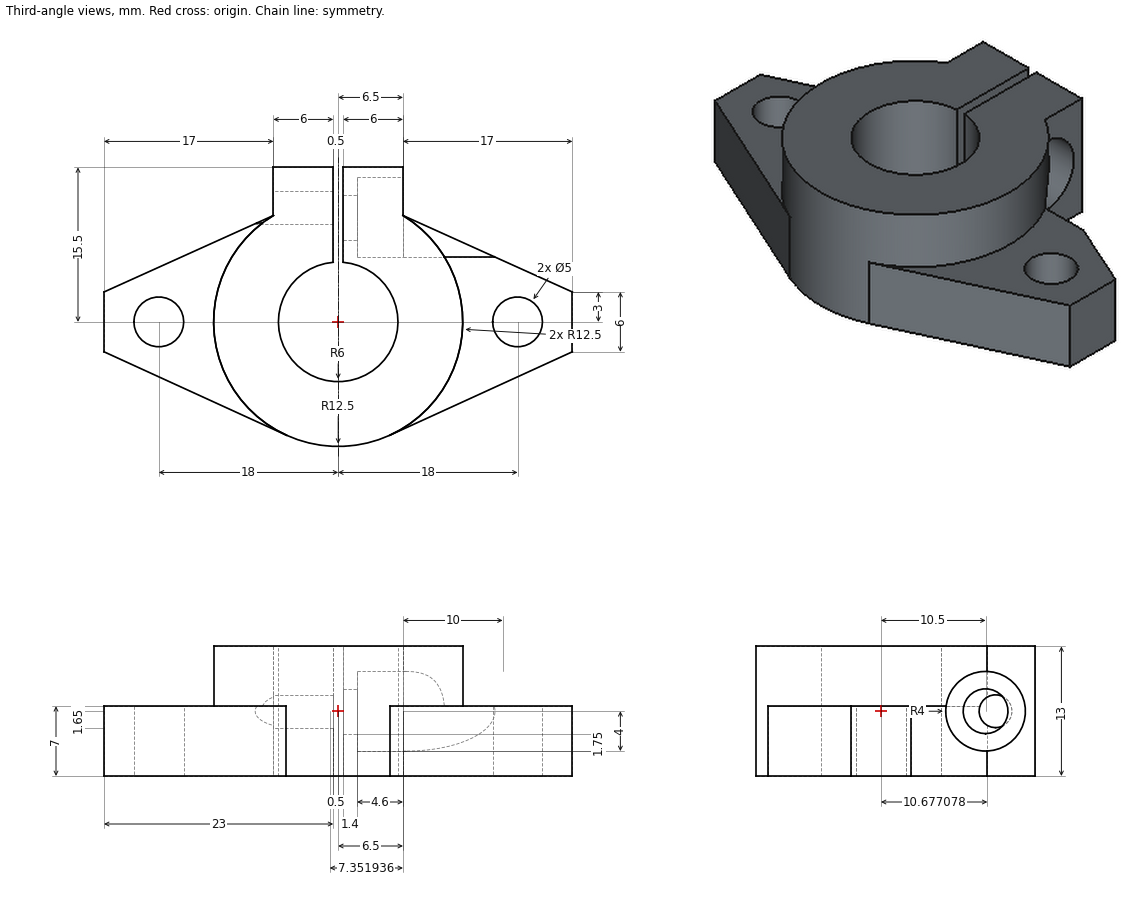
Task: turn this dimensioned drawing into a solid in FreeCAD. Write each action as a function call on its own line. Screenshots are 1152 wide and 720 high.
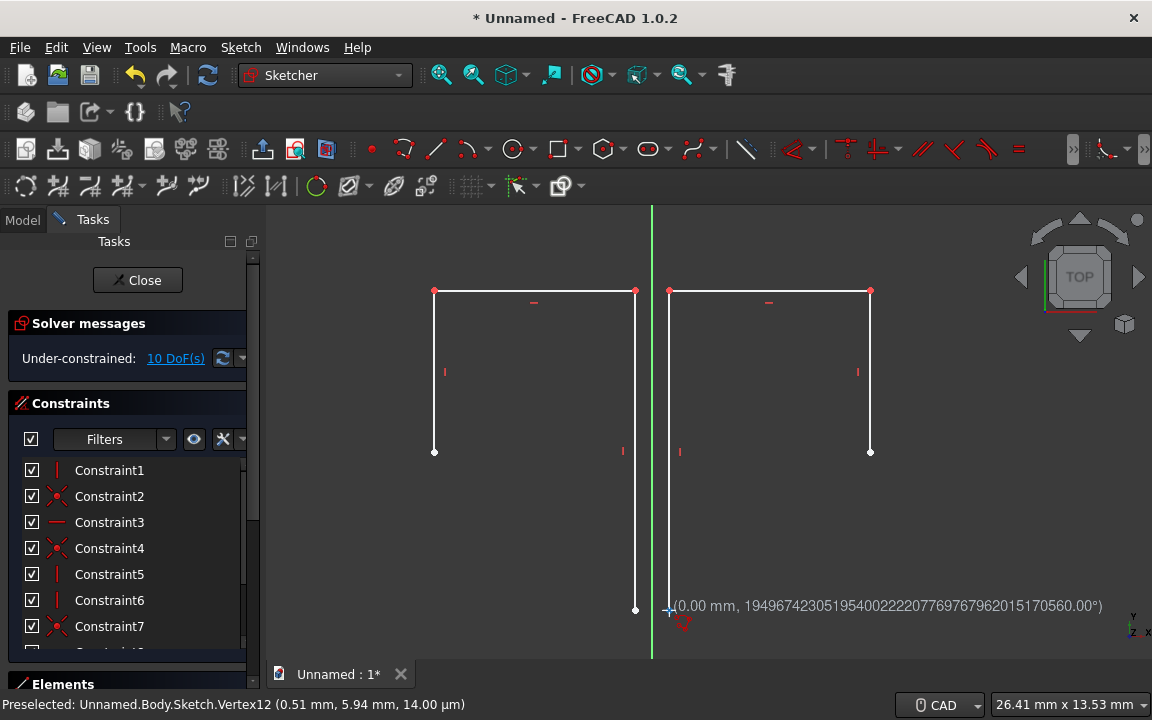
click(490, 150)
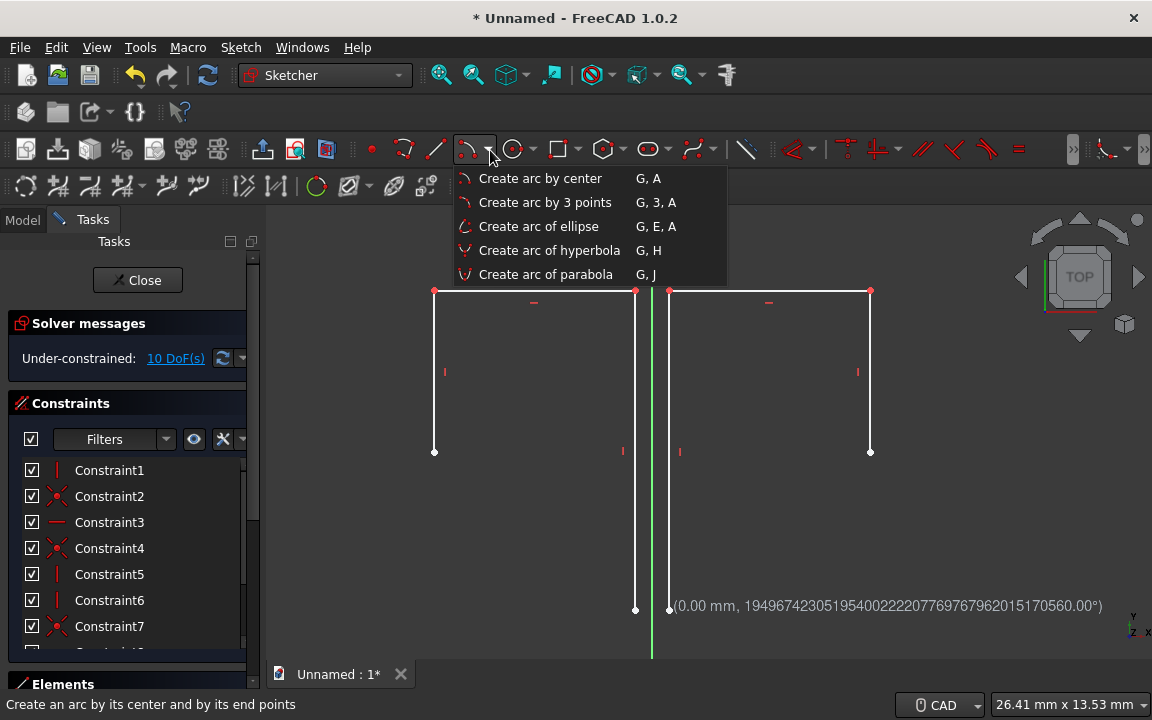
click(590, 202)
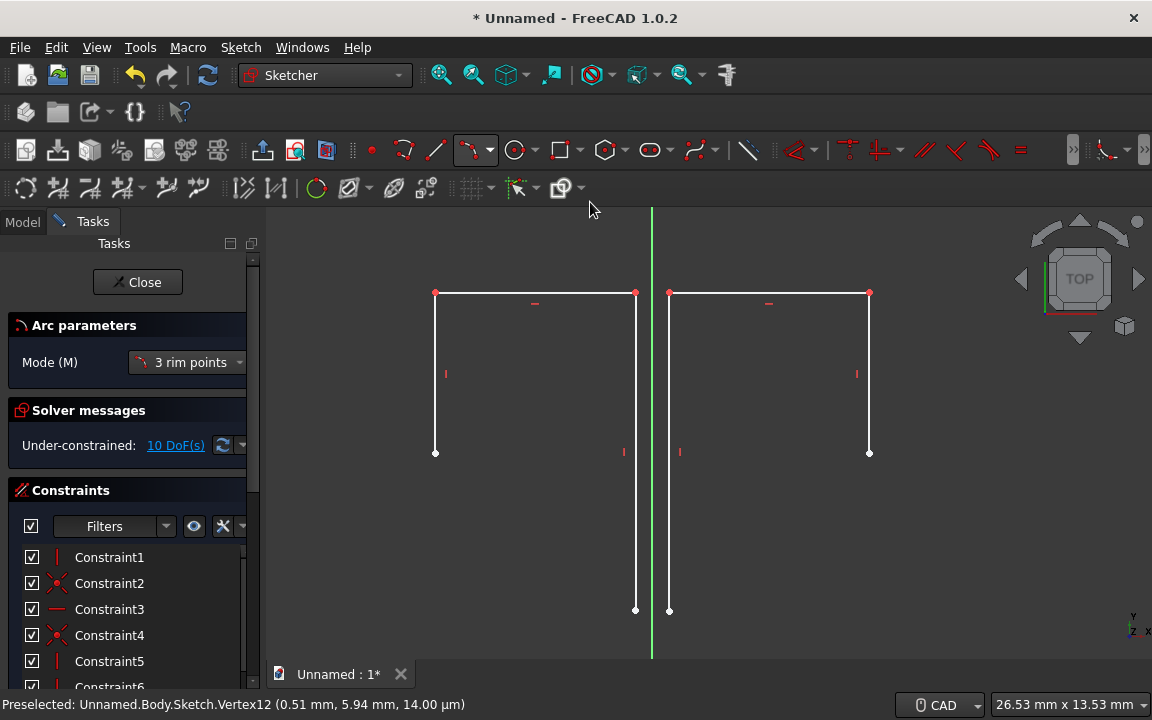
click(435, 454)
click(869, 454)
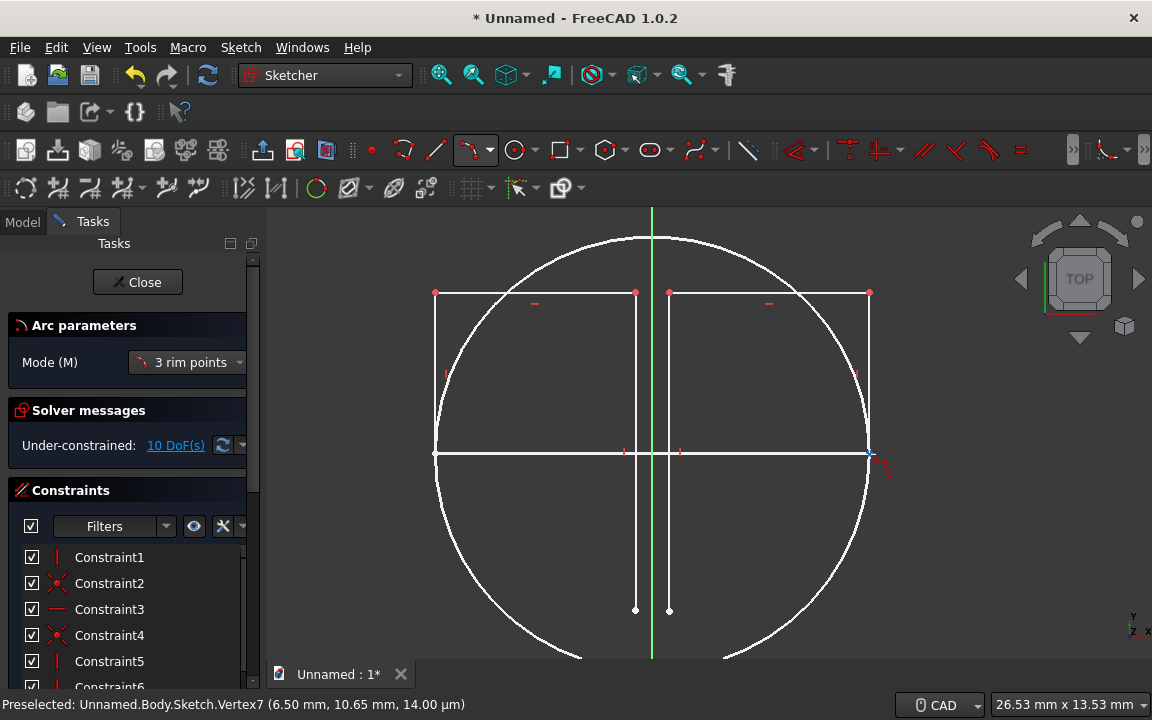
scroll(635, 292, down, 6)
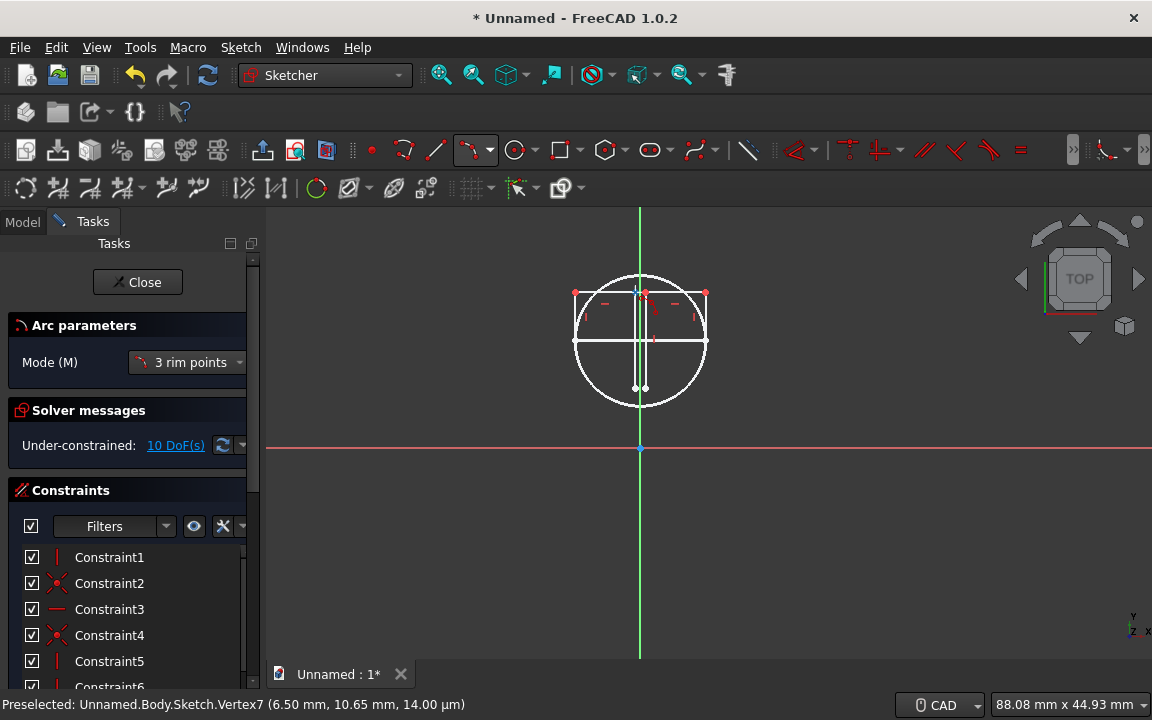
click(578, 557)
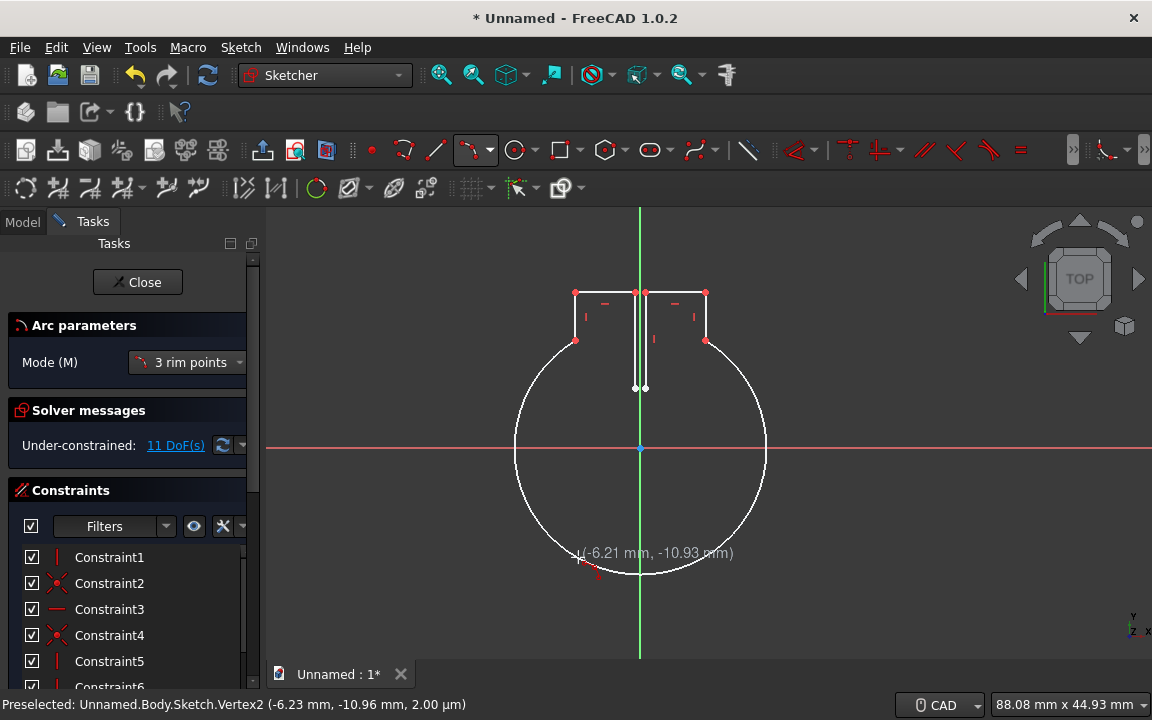
scroll(645, 388, up, 6)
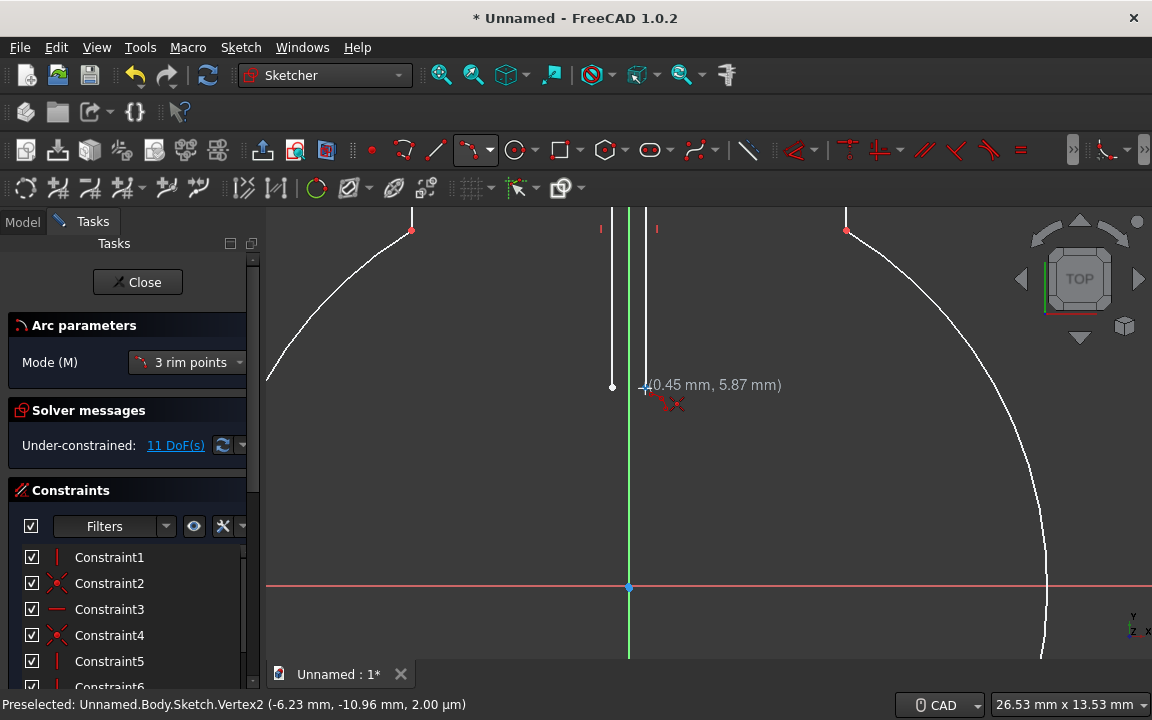
click(646, 388)
click(612, 388)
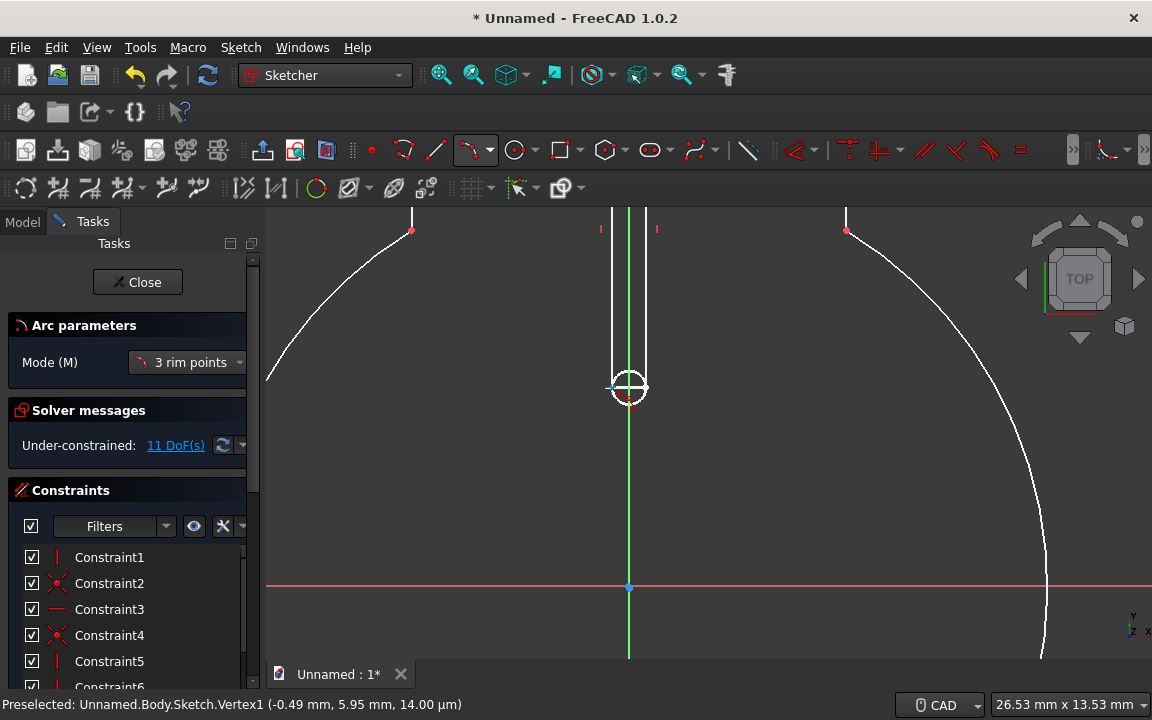
scroll(645, 388, down, 6)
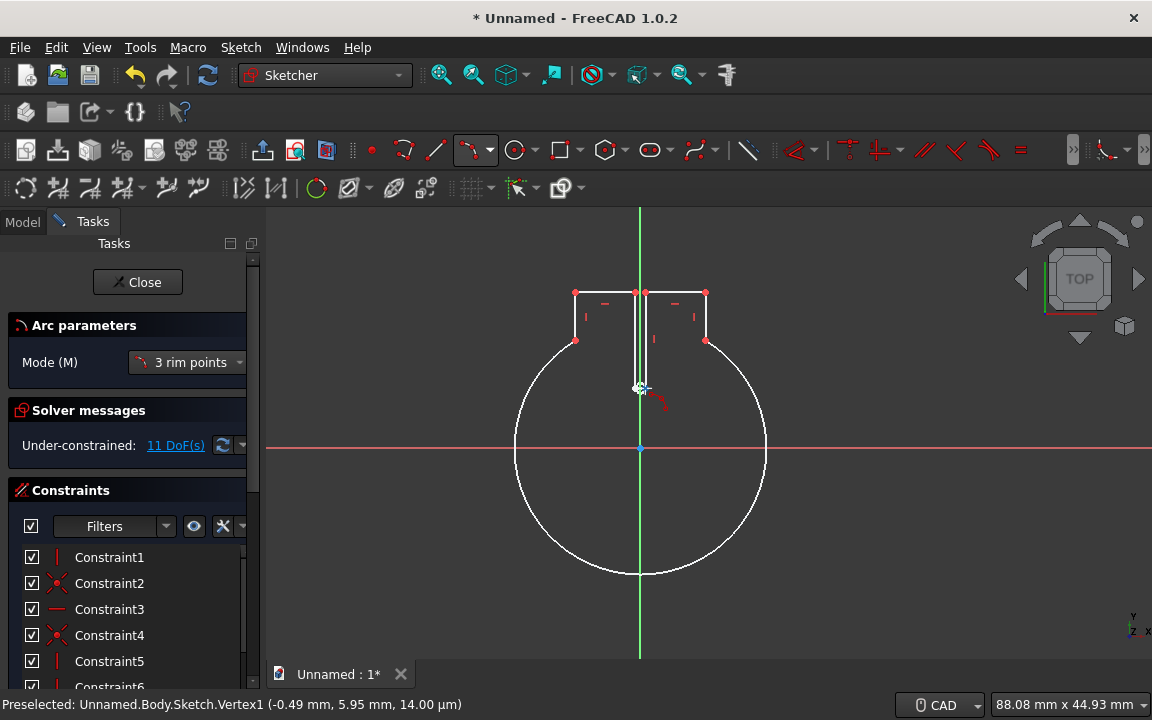
click(606, 497)
key(Escape)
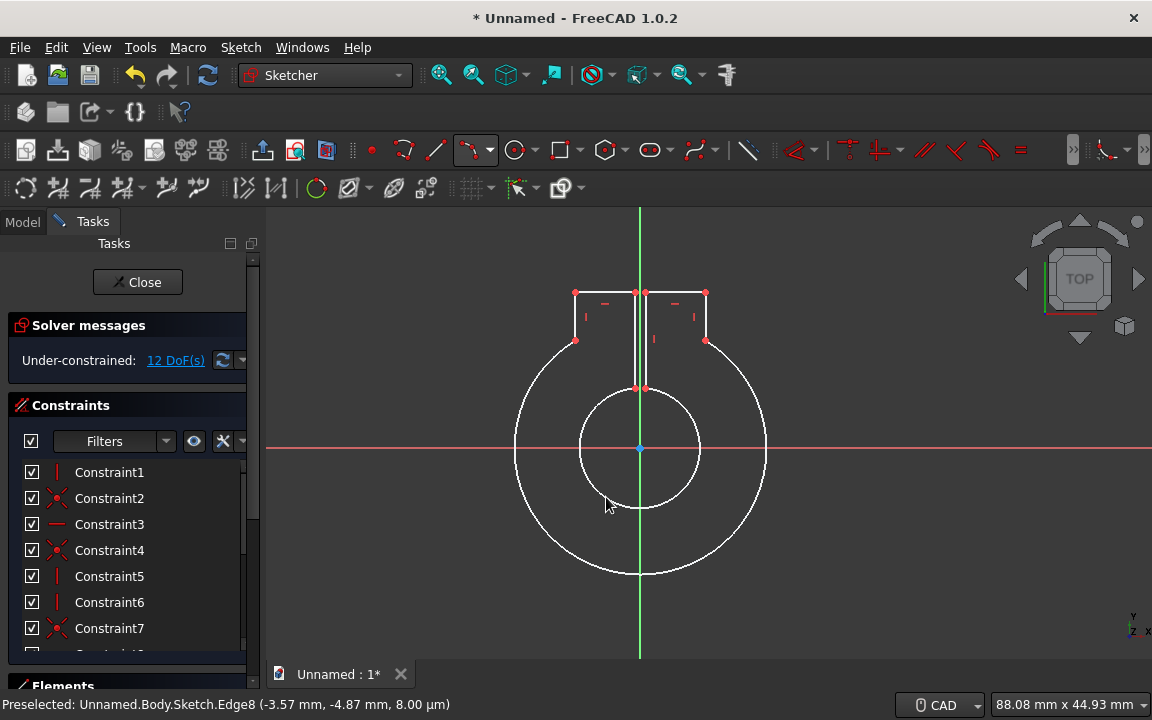
click(532, 513)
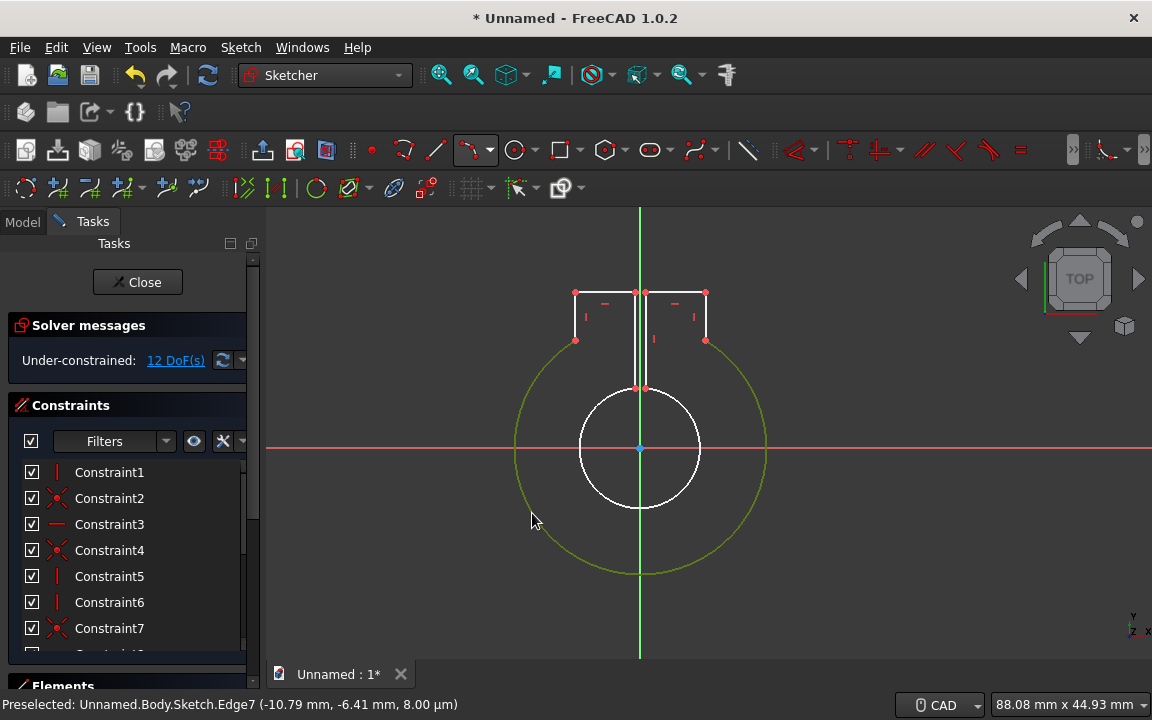
click(583, 468)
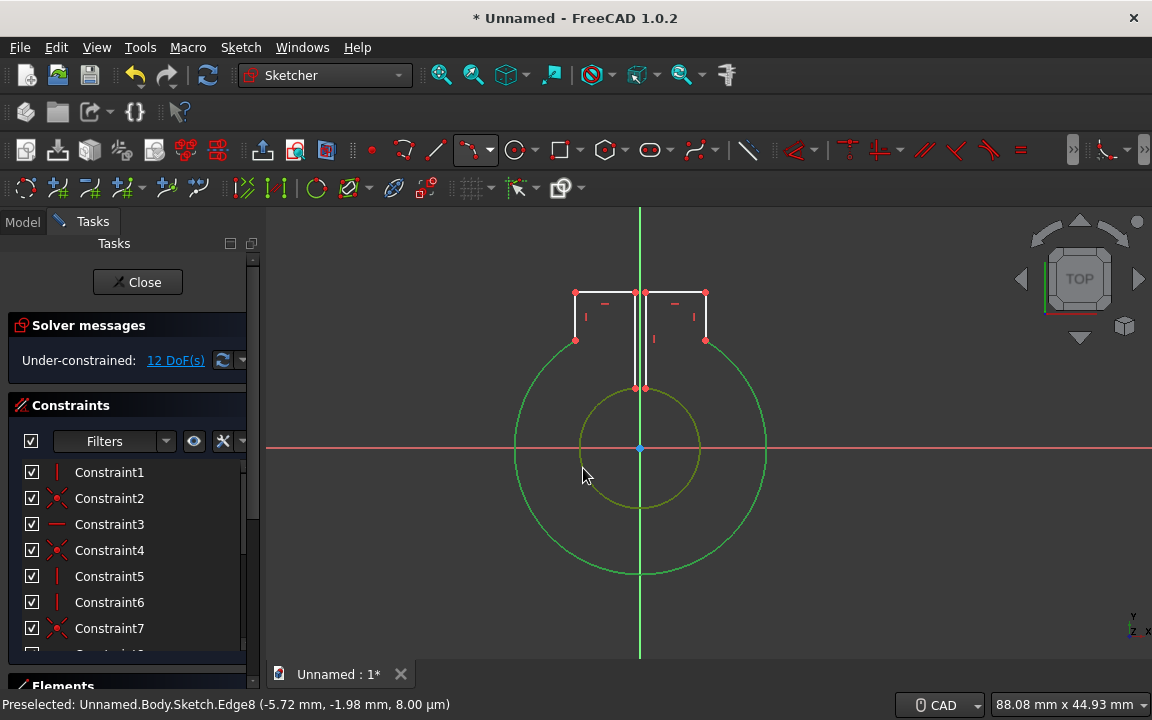
click(848, 150)